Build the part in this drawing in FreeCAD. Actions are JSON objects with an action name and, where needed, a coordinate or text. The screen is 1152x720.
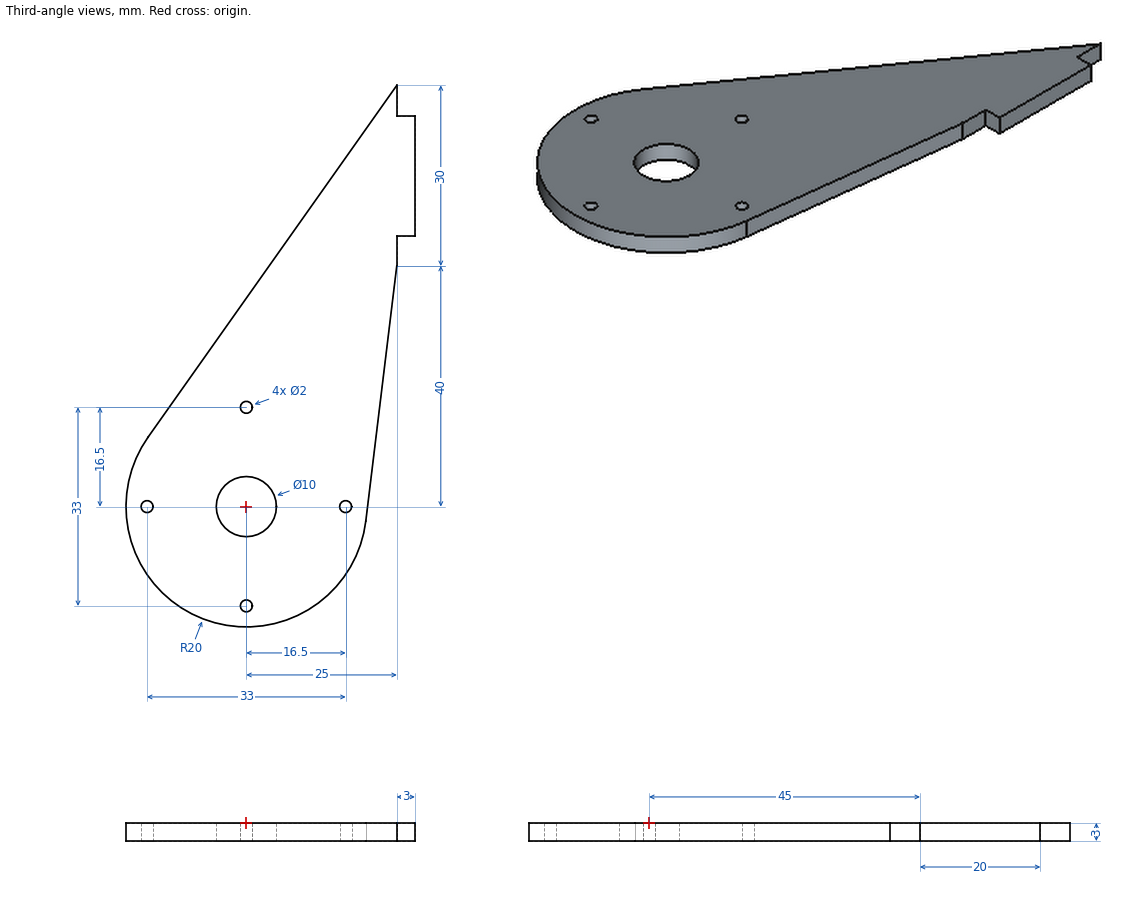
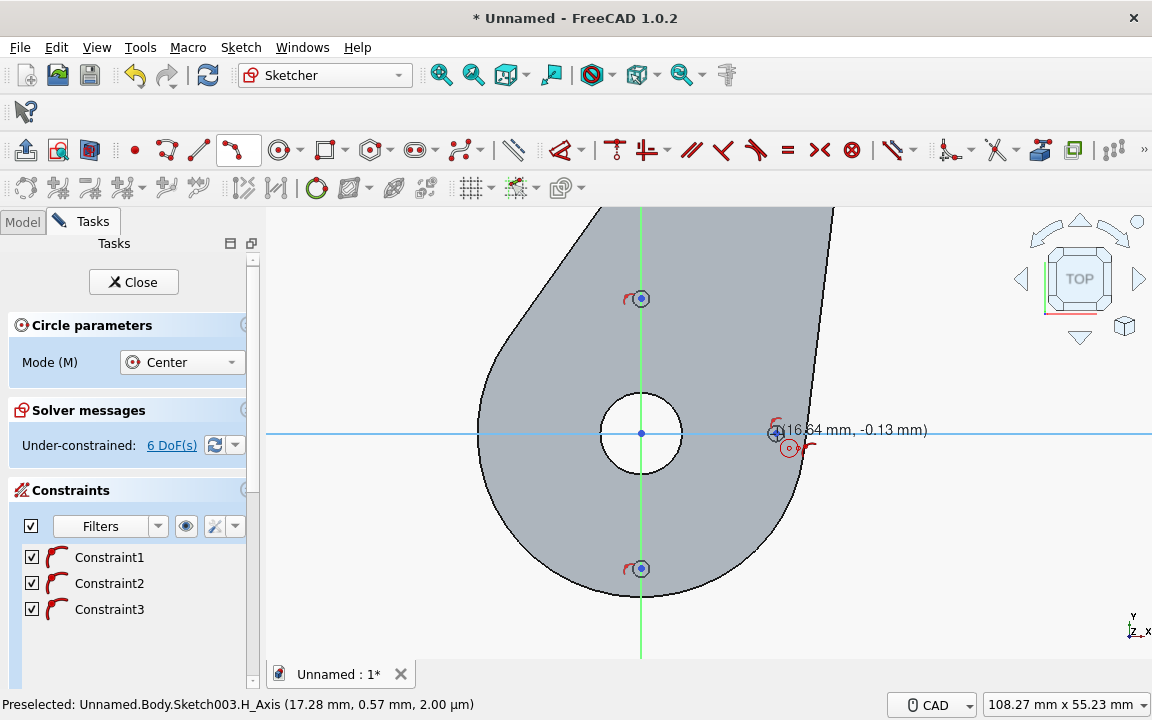
{"action": "scroll", "coordinate": [506, 434], "scroll_direction": "up", "scroll_amount": 6}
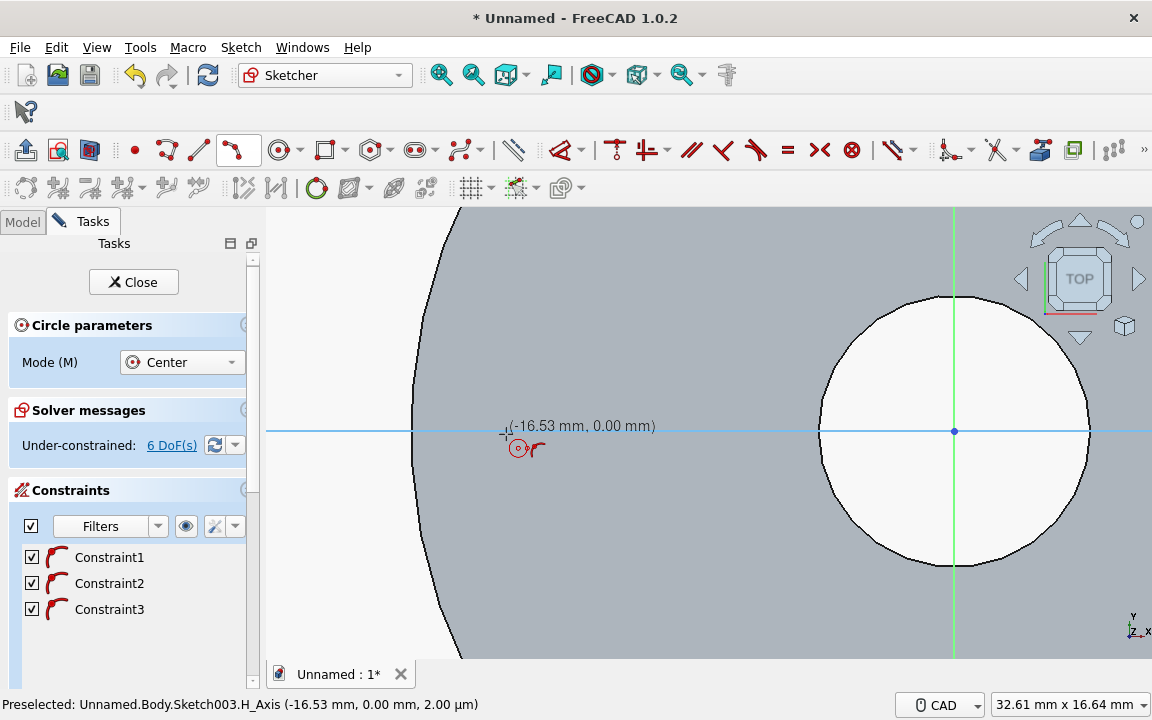
{"action": "left_click", "coordinate": [506, 431]}
{"action": "left_click", "coordinate": [525, 412]}
{"action": "key", "text": "Escape"}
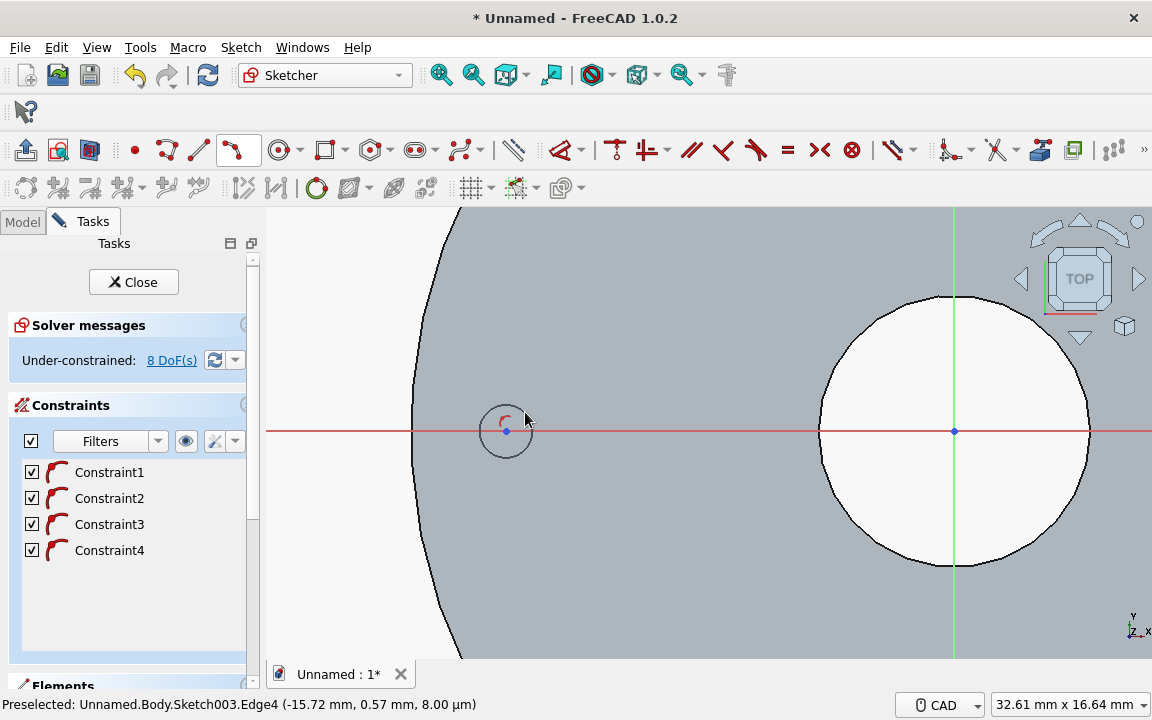
{"action": "scroll", "coordinate": [505, 434], "scroll_direction": "down", "scroll_amount": 6}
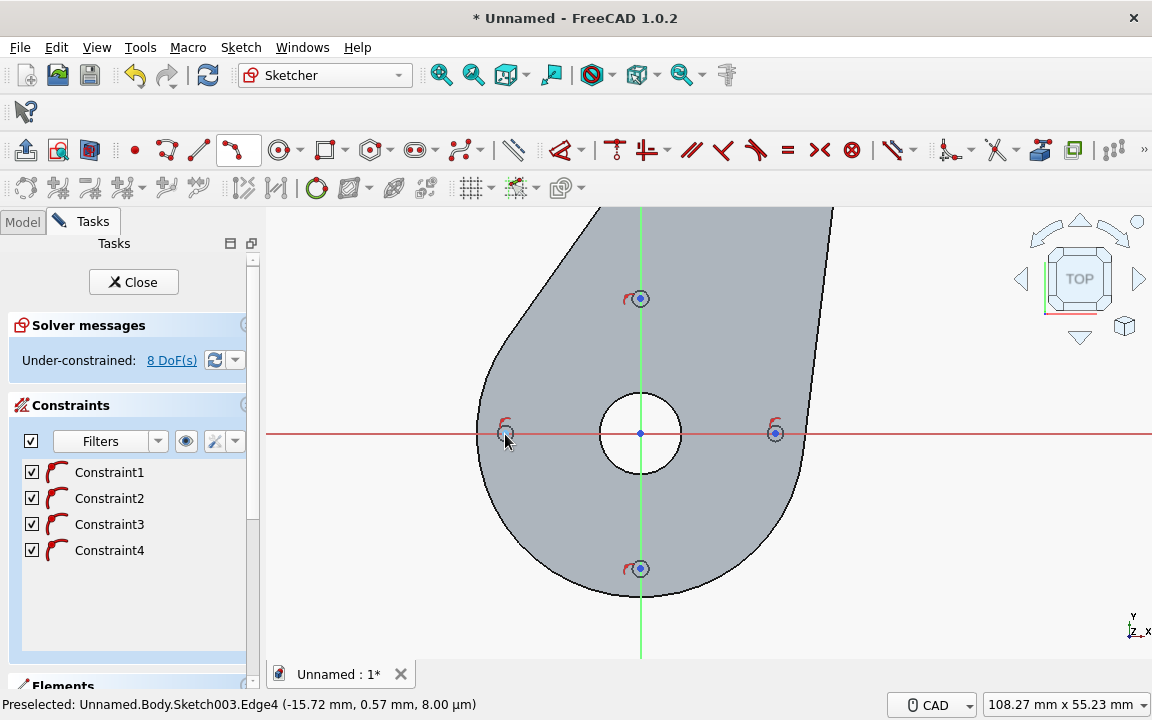
{"action": "scroll", "coordinate": [646, 293], "scroll_direction": "up", "scroll_amount": 5}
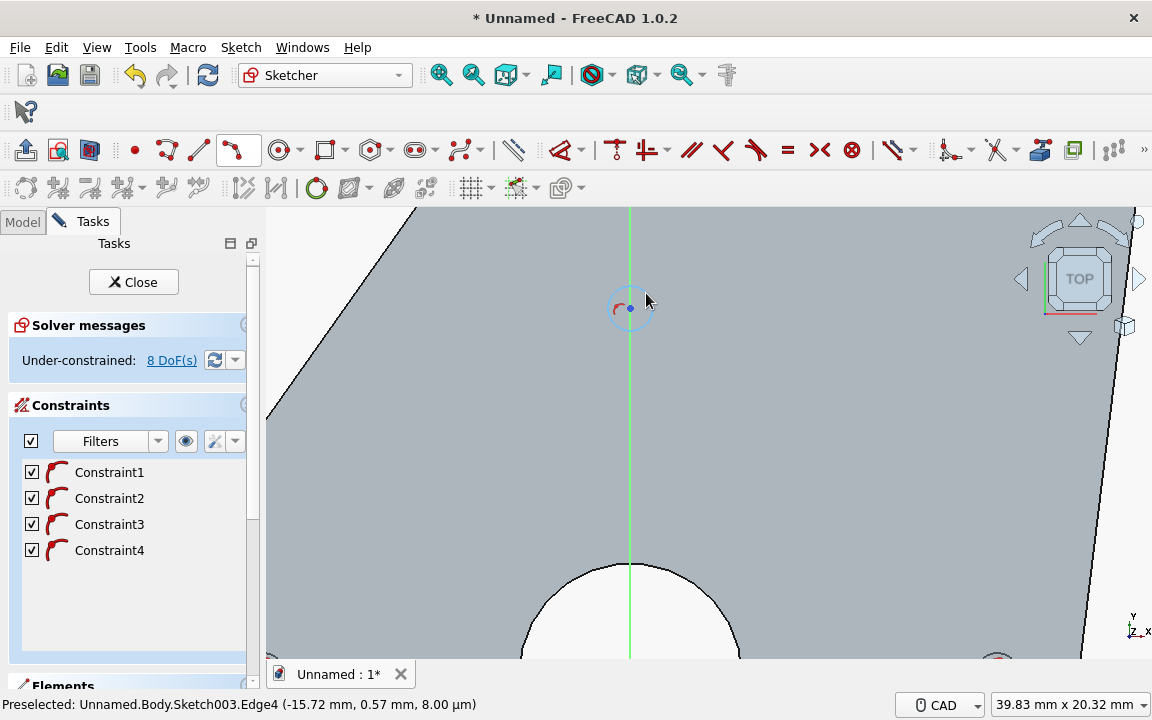
{"action": "left_click", "coordinate": [646, 293]}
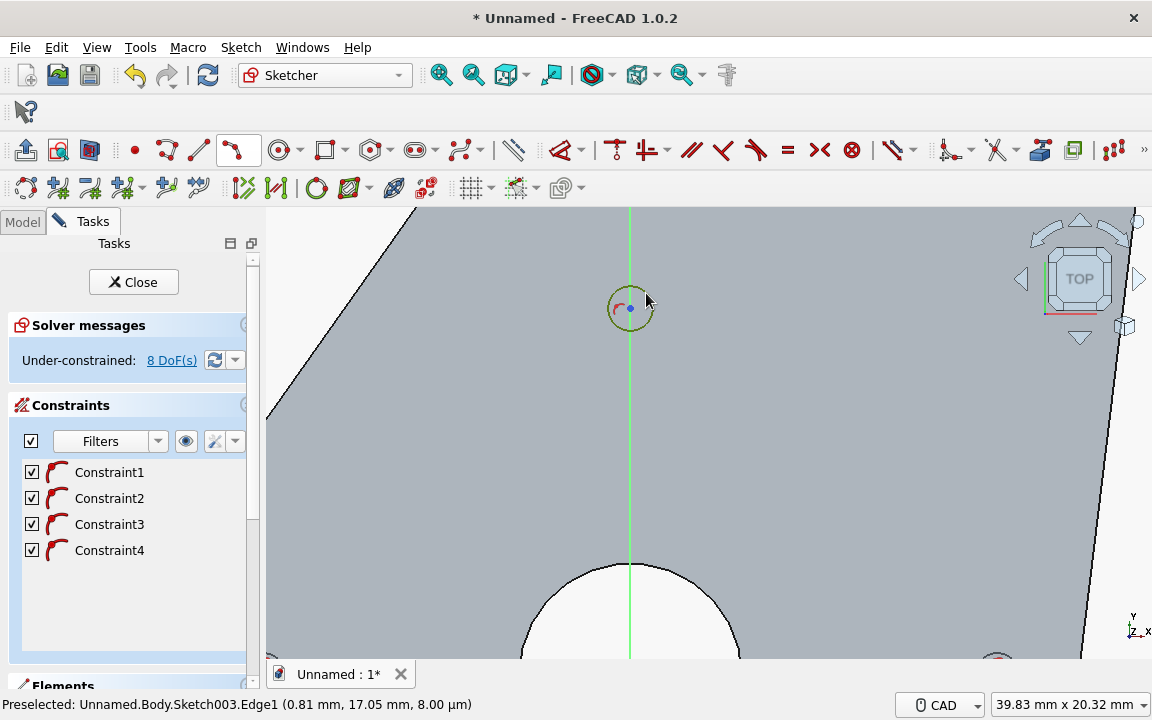
{"action": "scroll", "coordinate": [646, 292], "scroll_direction": "down", "scroll_amount": 5}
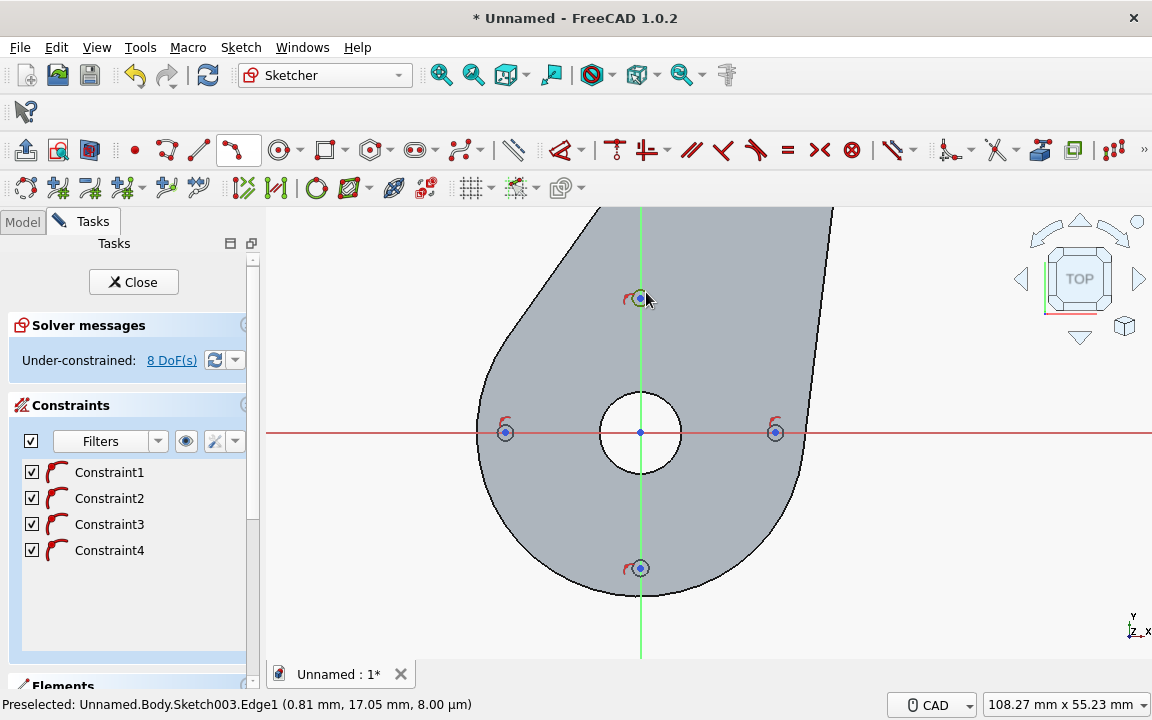
{"action": "scroll", "coordinate": [646, 563], "scroll_direction": "up", "scroll_amount": 5}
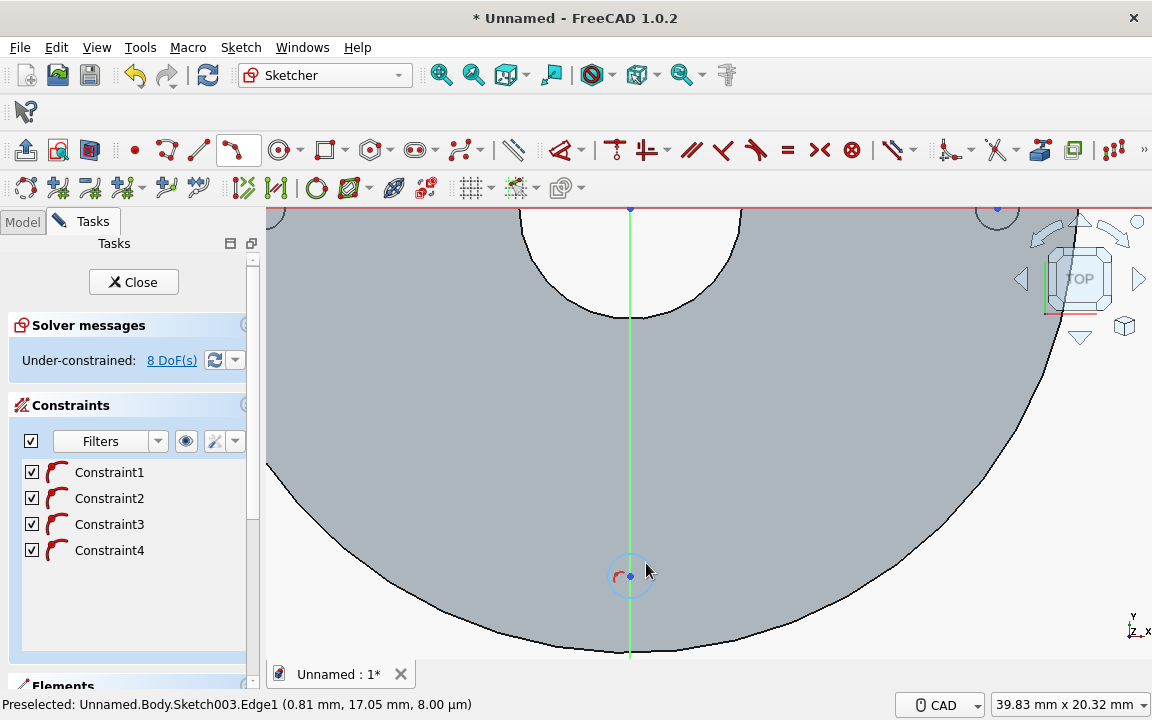
{"action": "left_click", "coordinate": [646, 560]}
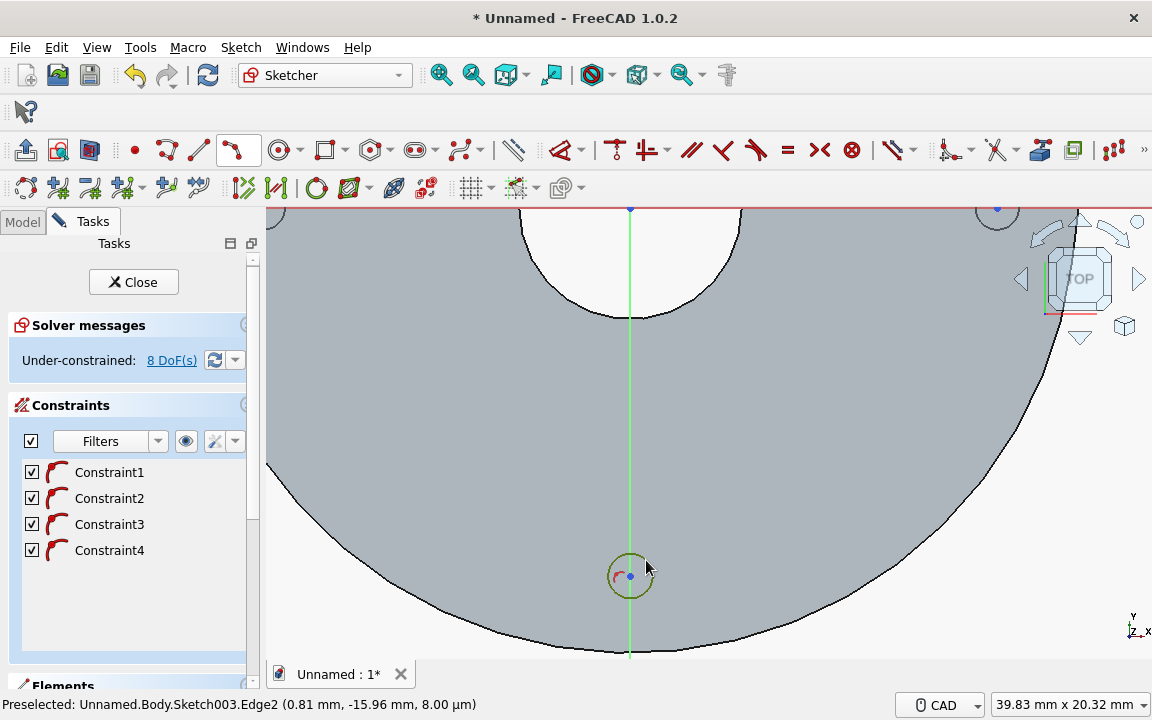
{"action": "scroll", "coordinate": [646, 564], "scroll_direction": "down", "scroll_amount": 5}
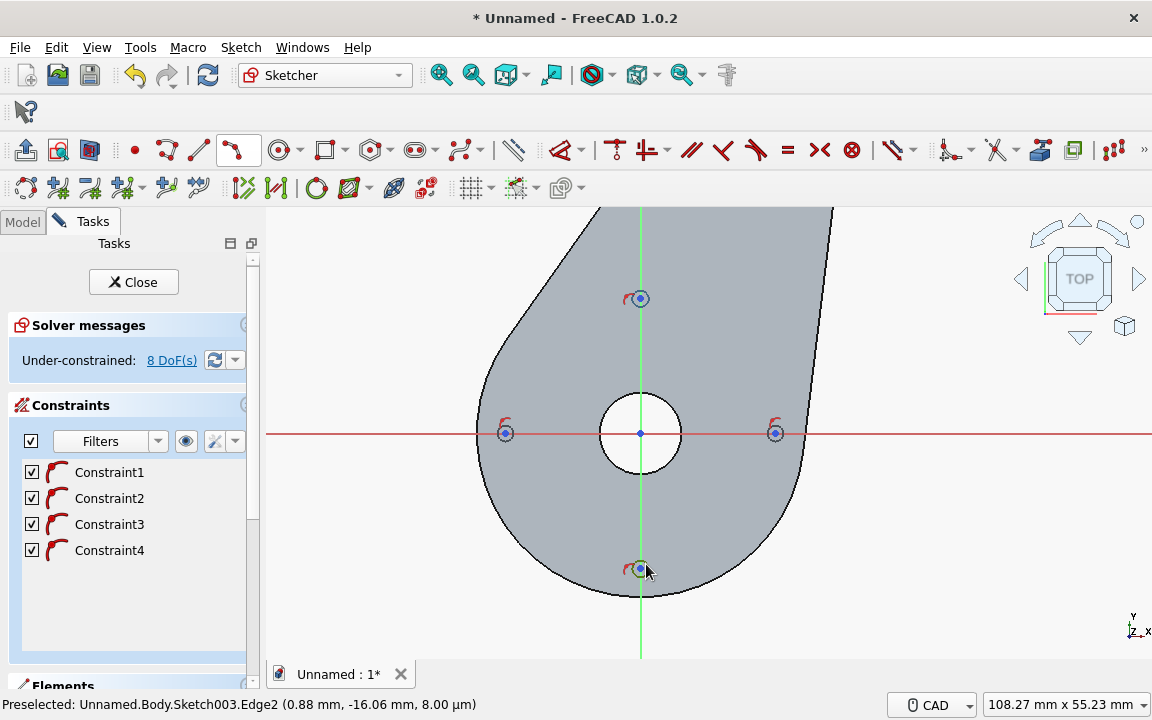
{"action": "scroll", "coordinate": [781, 428], "scroll_direction": "up", "scroll_amount": 5}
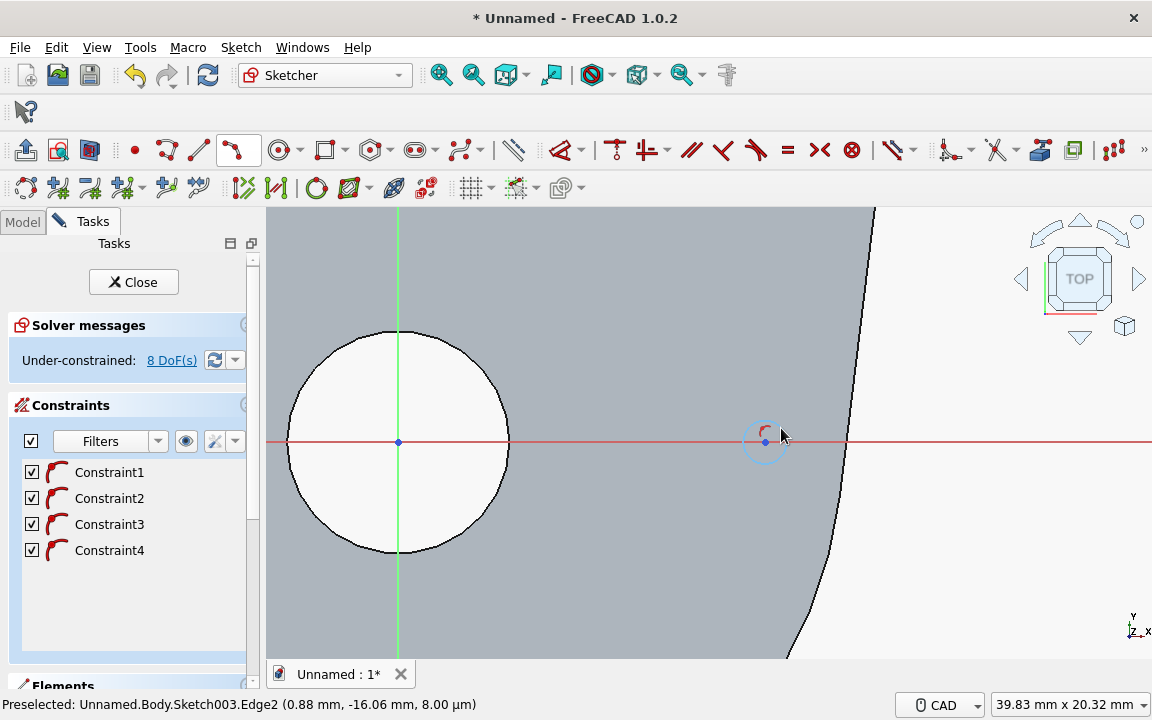
{"action": "left_click", "coordinate": [780, 427]}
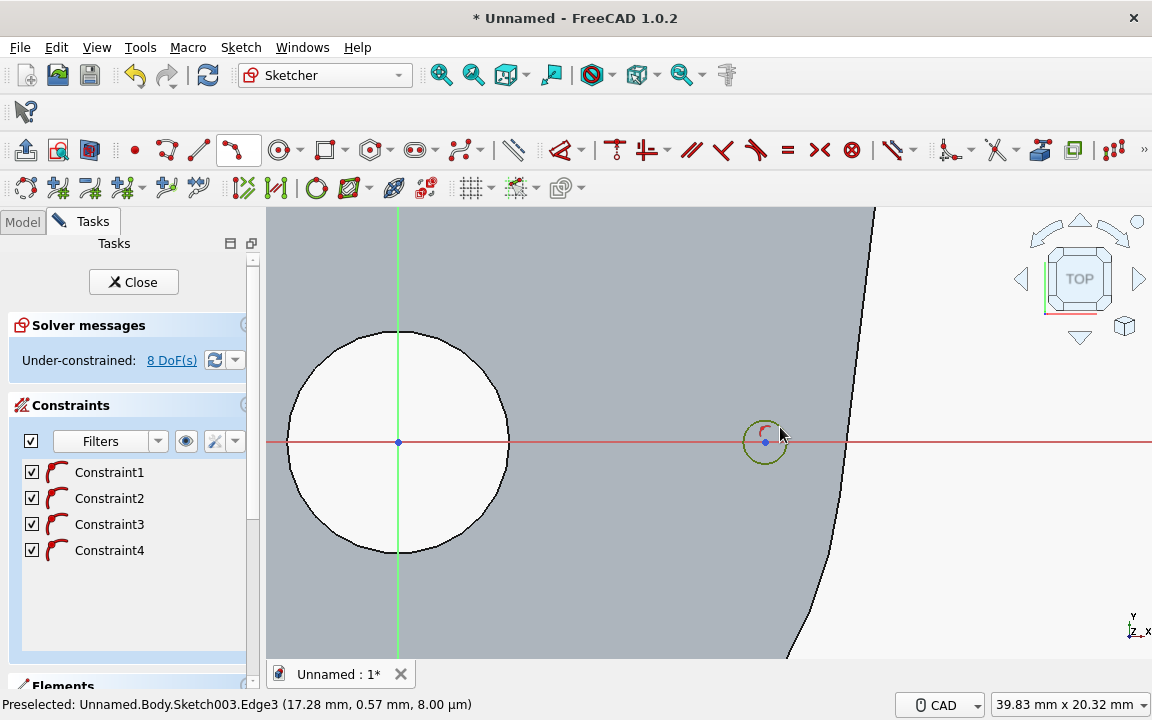
{"action": "scroll", "coordinate": [781, 428], "scroll_direction": "down", "scroll_amount": 5}